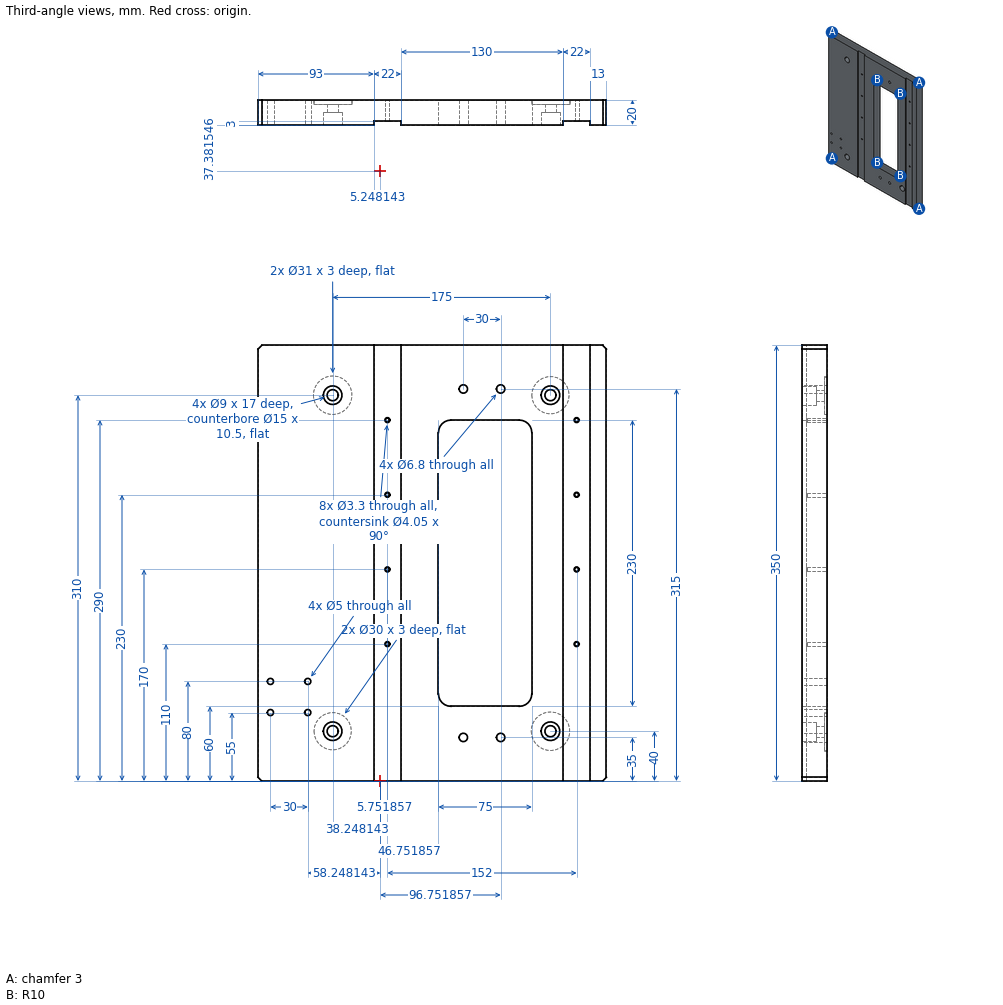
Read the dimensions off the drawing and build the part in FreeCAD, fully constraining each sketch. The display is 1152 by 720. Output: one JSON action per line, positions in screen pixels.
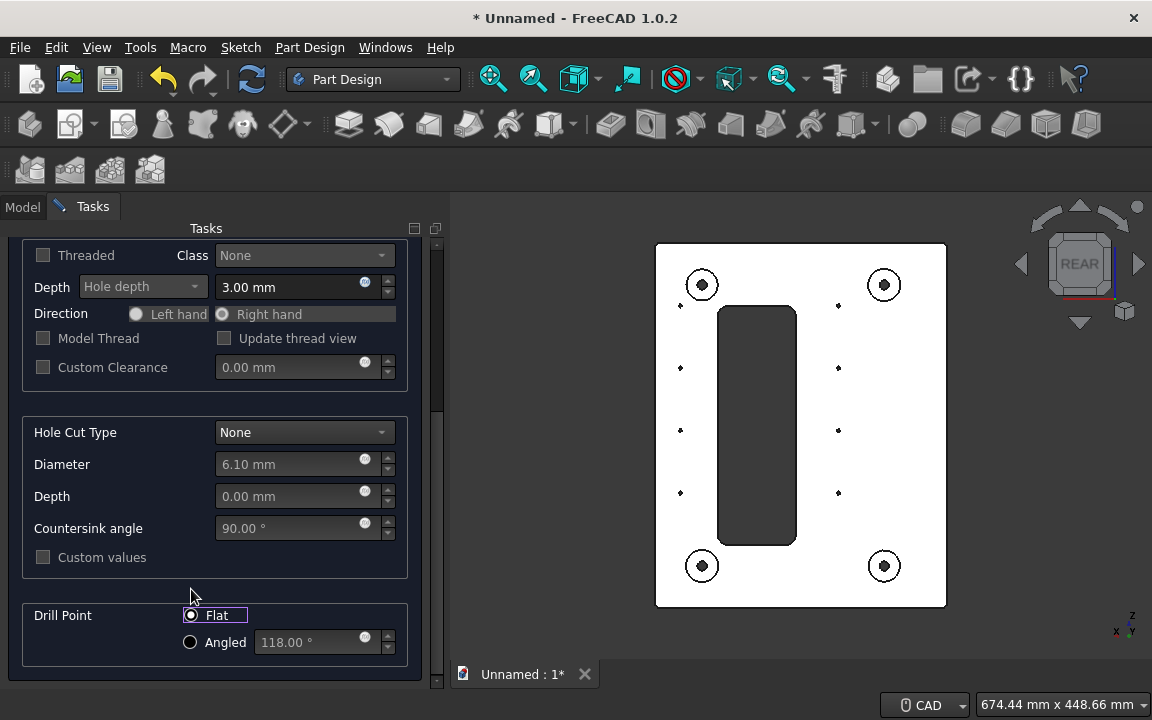
{"action": "scroll", "coordinate": [437, 463], "scroll_direction": "up", "scroll_amount": 6}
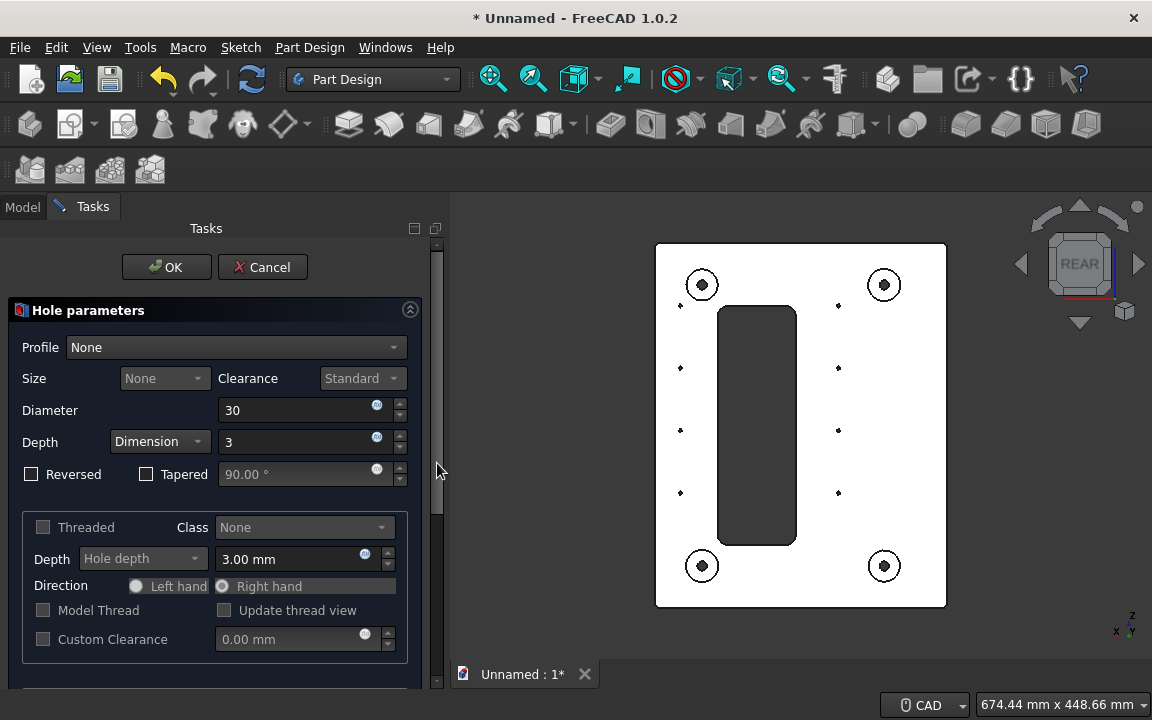
{"action": "left_click", "coordinate": [167, 267]}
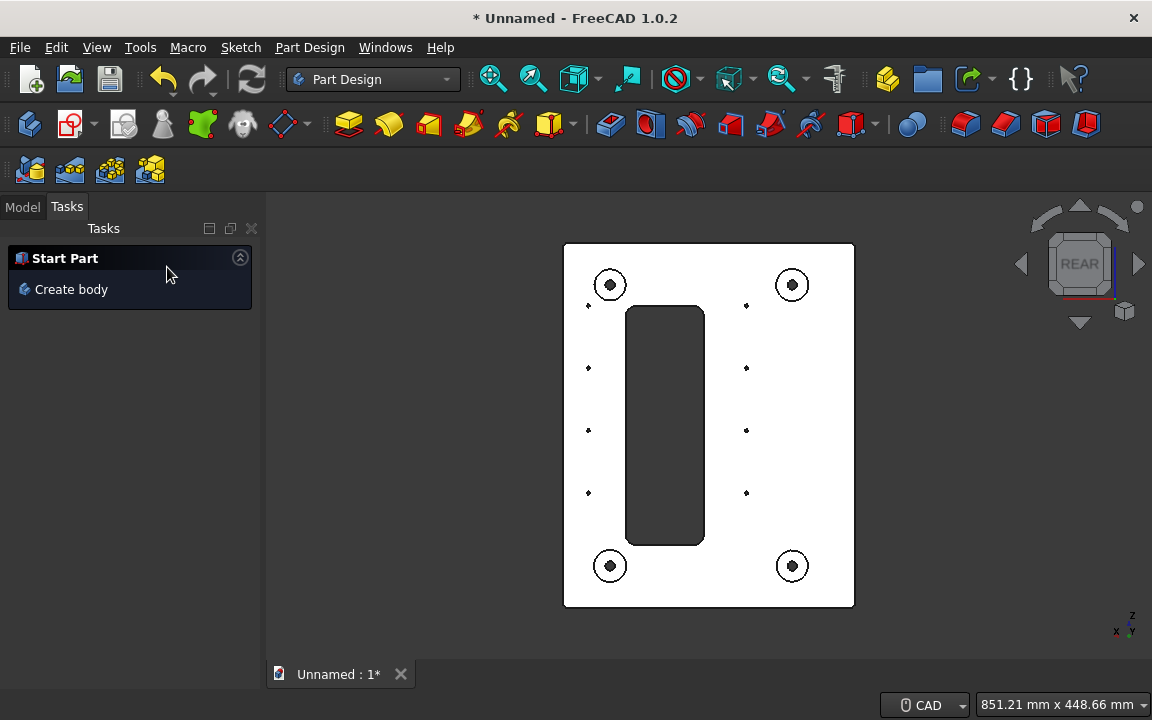
{"action": "left_click", "coordinate": [792, 477]}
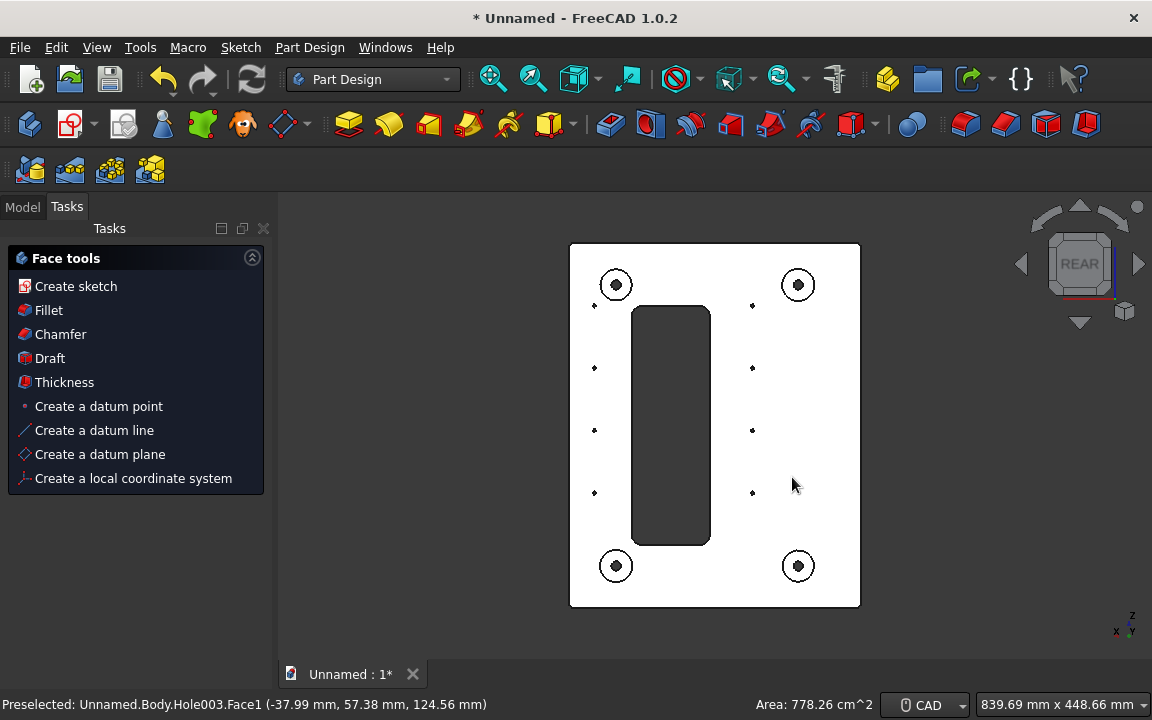
{"action": "left_click", "coordinate": [70, 124]}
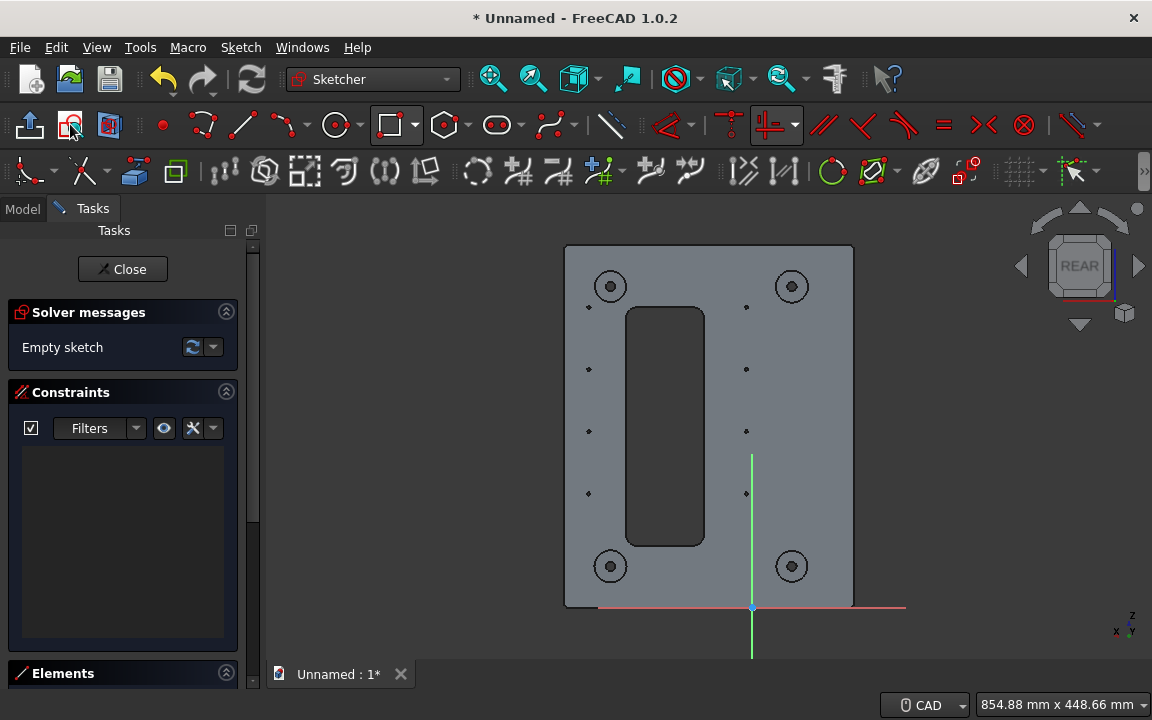
{"action": "scroll", "coordinate": [370, 353], "scroll_direction": "down", "scroll_amount": 1}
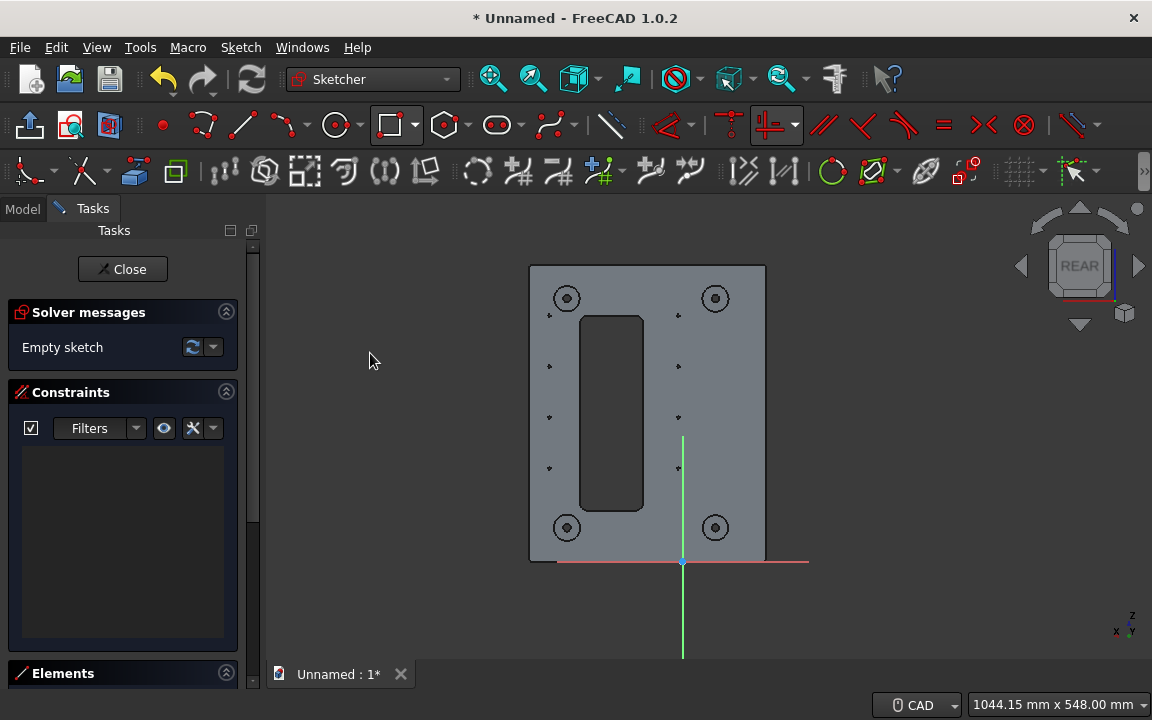
{"action": "left_click", "coordinate": [336, 126]}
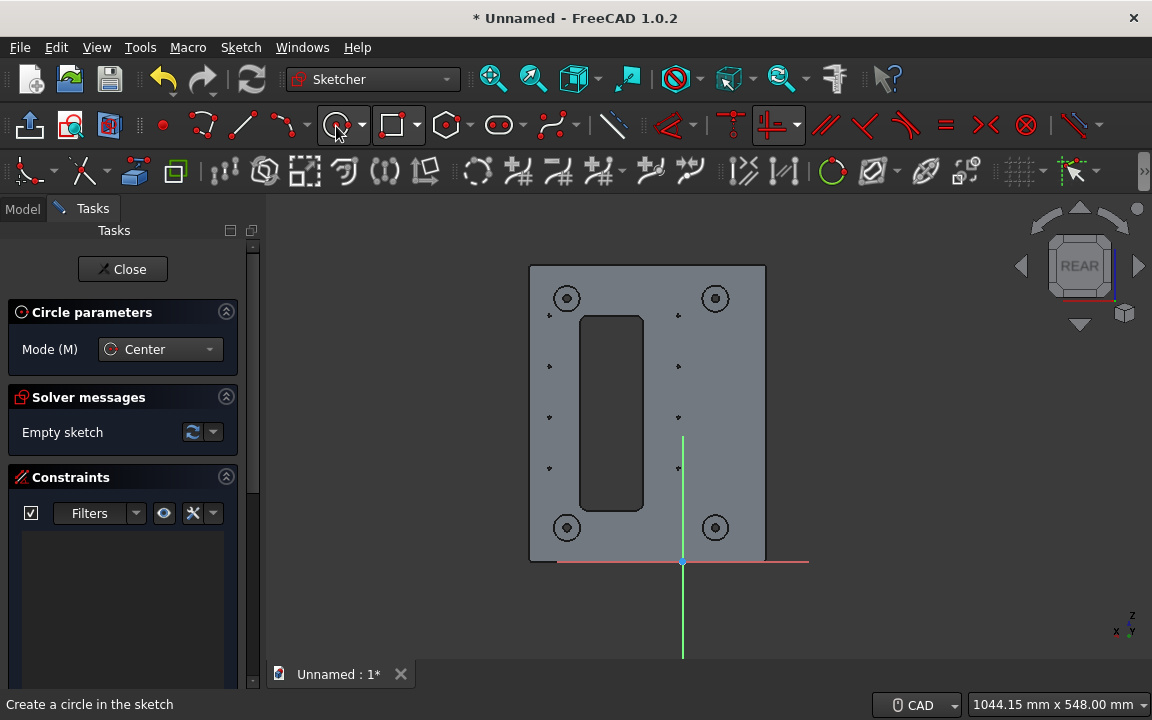
{"action": "scroll", "coordinate": [601, 294], "scroll_direction": "up", "scroll_amount": 11}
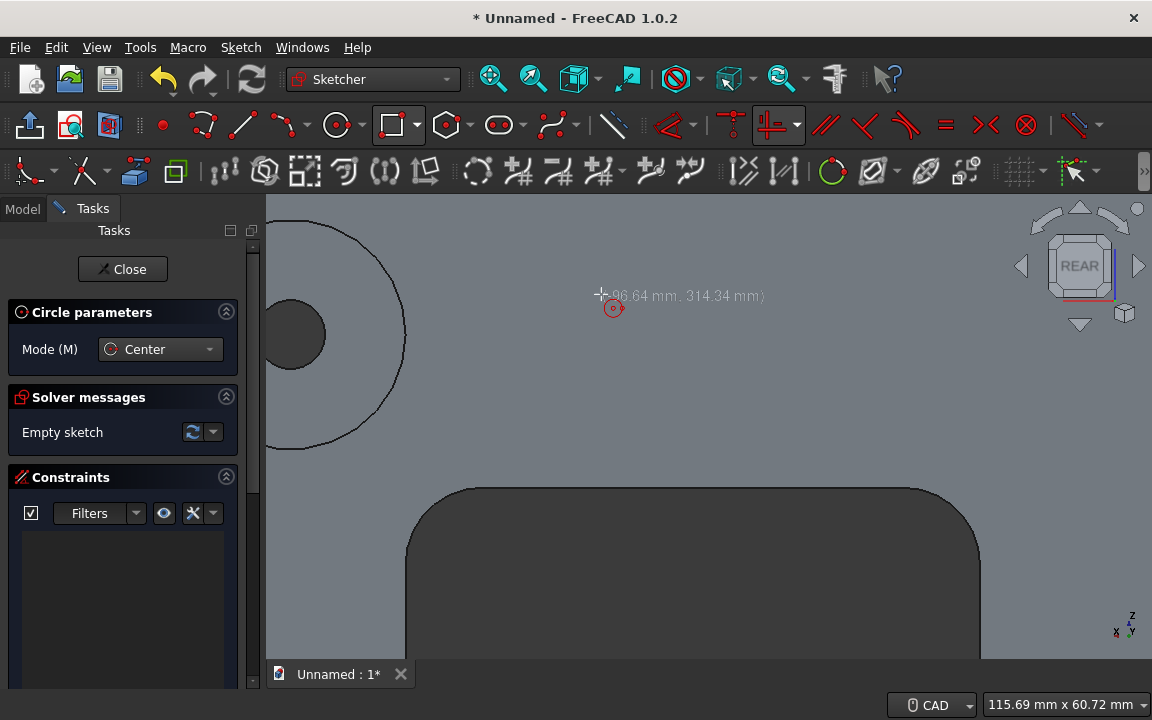
{"action": "scroll", "coordinate": [601, 294], "scroll_direction": "down", "scroll_amount": 11}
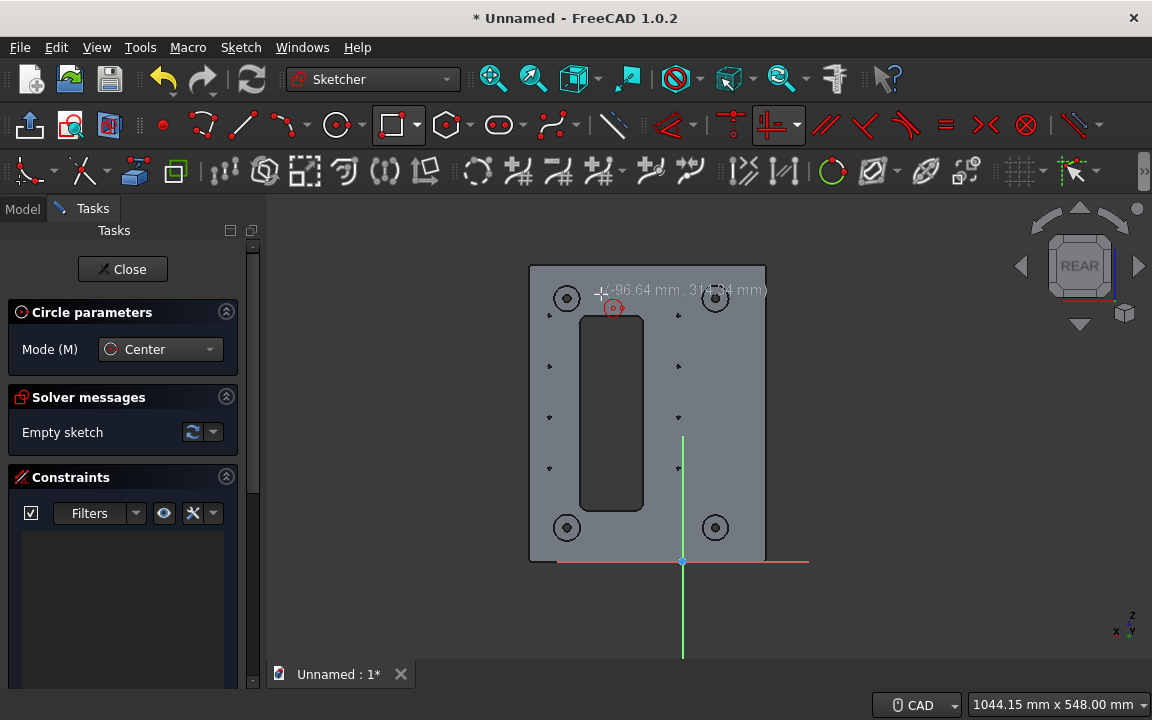
{"action": "left_click", "coordinate": [601, 294]}
{"action": "mouse_move", "coordinate": [603, 292]}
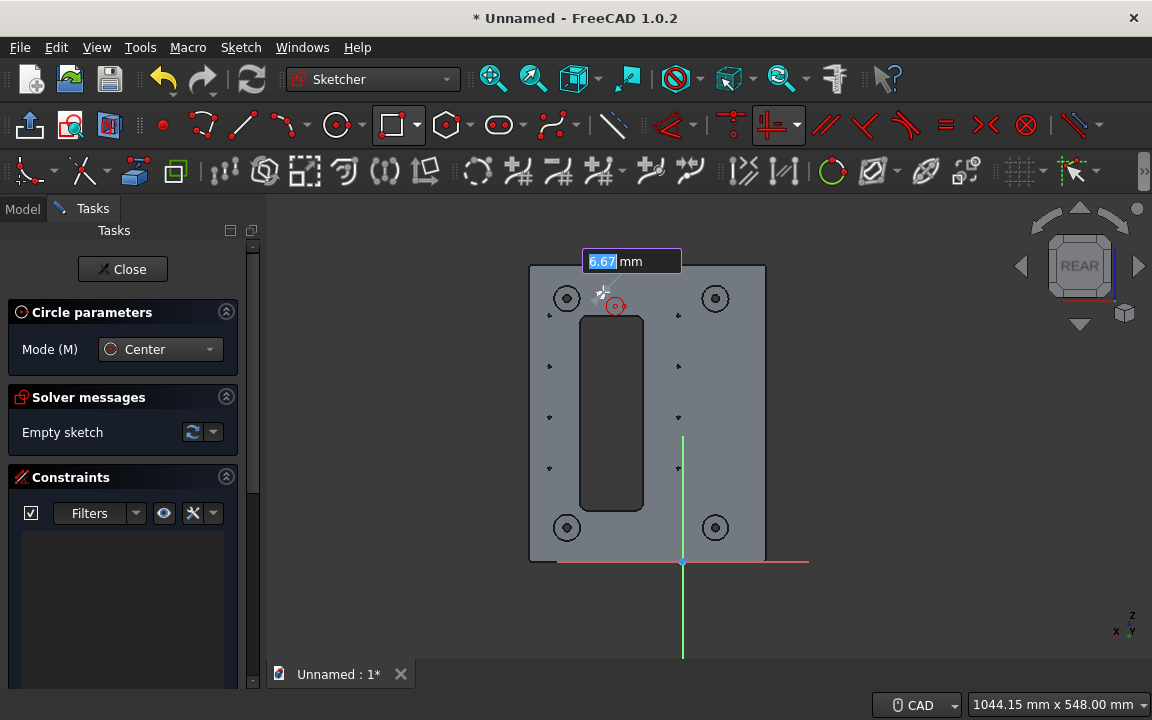
{"action": "type", "text": "6.8"}
{"action": "key", "text": "Return"}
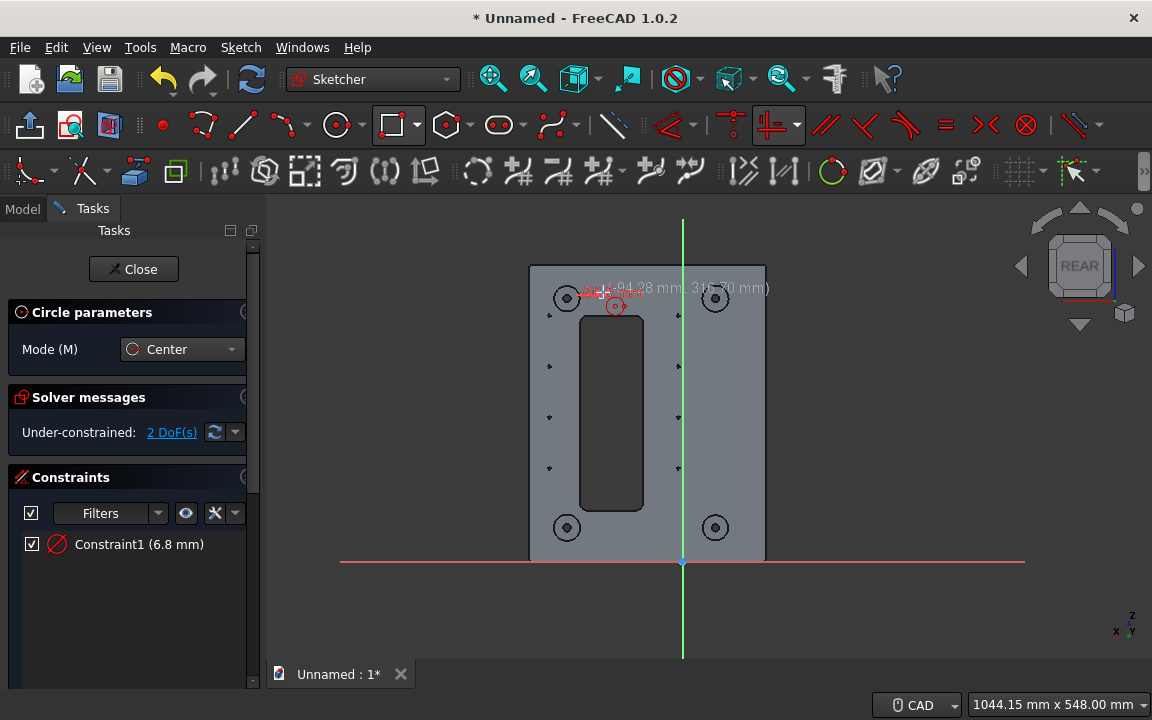
{"action": "scroll", "coordinate": [626, 294], "scroll_direction": "up", "scroll_amount": 11}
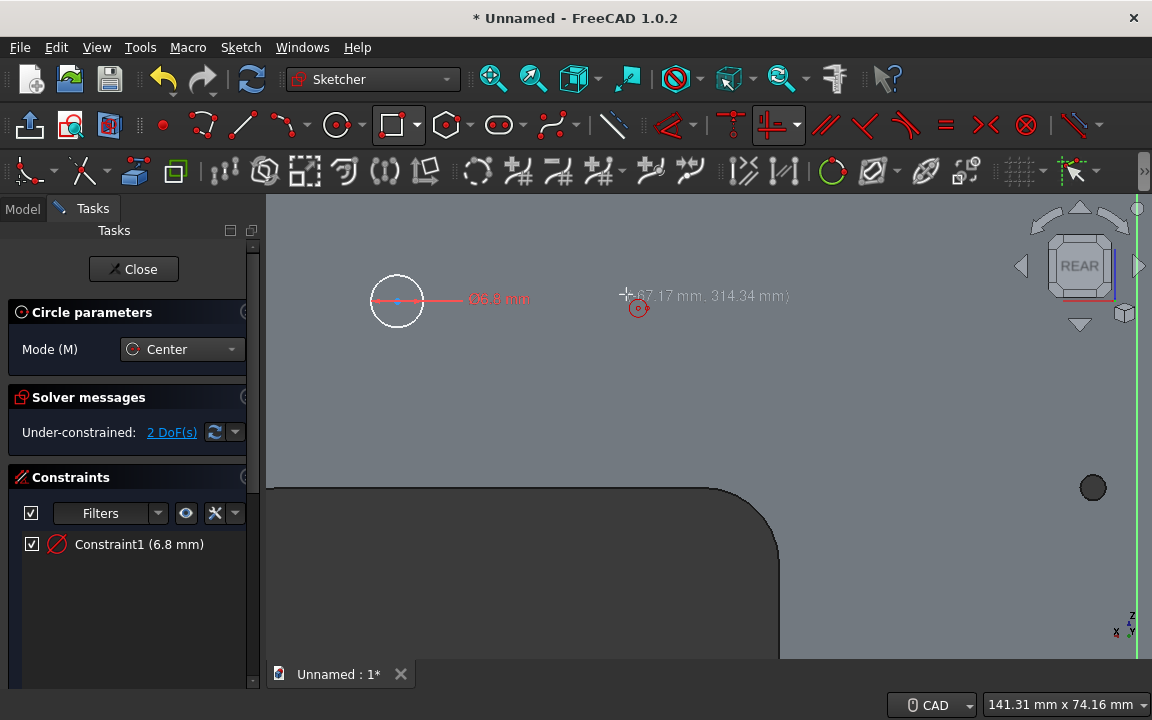
{"action": "scroll", "coordinate": [626, 294], "scroll_direction": "down", "scroll_amount": 11}